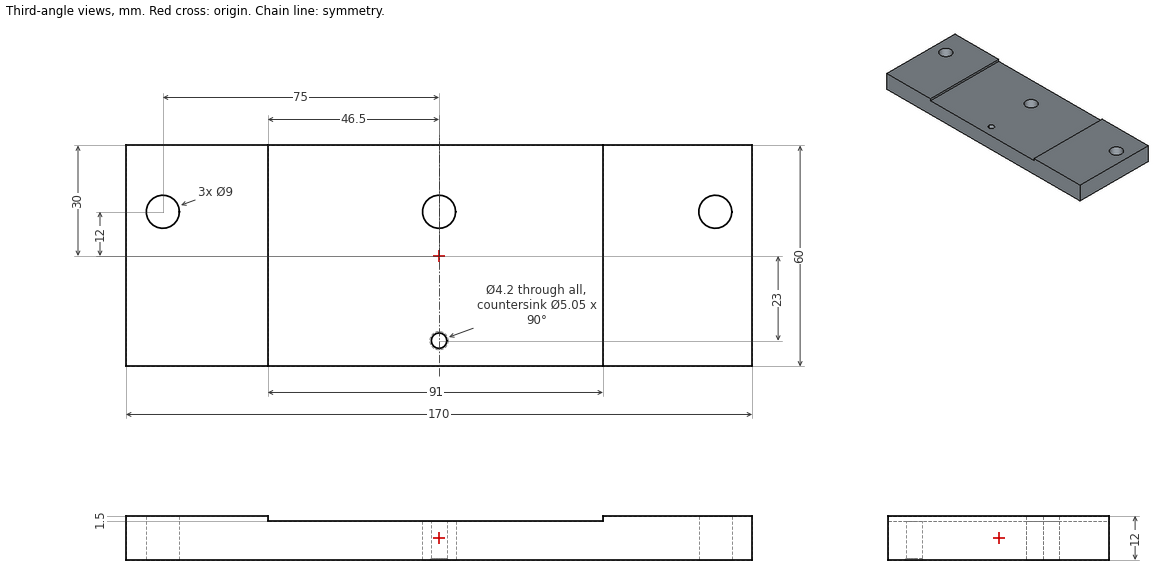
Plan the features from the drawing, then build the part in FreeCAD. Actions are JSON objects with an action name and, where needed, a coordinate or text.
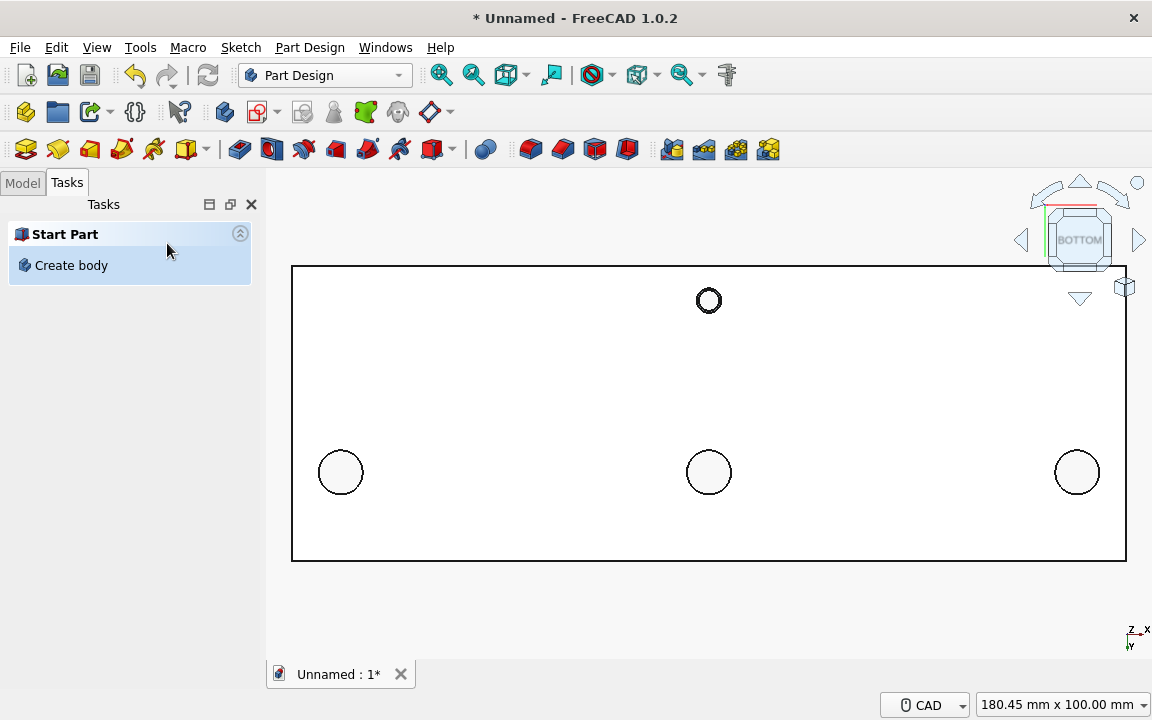
{"action": "key", "text": "0"}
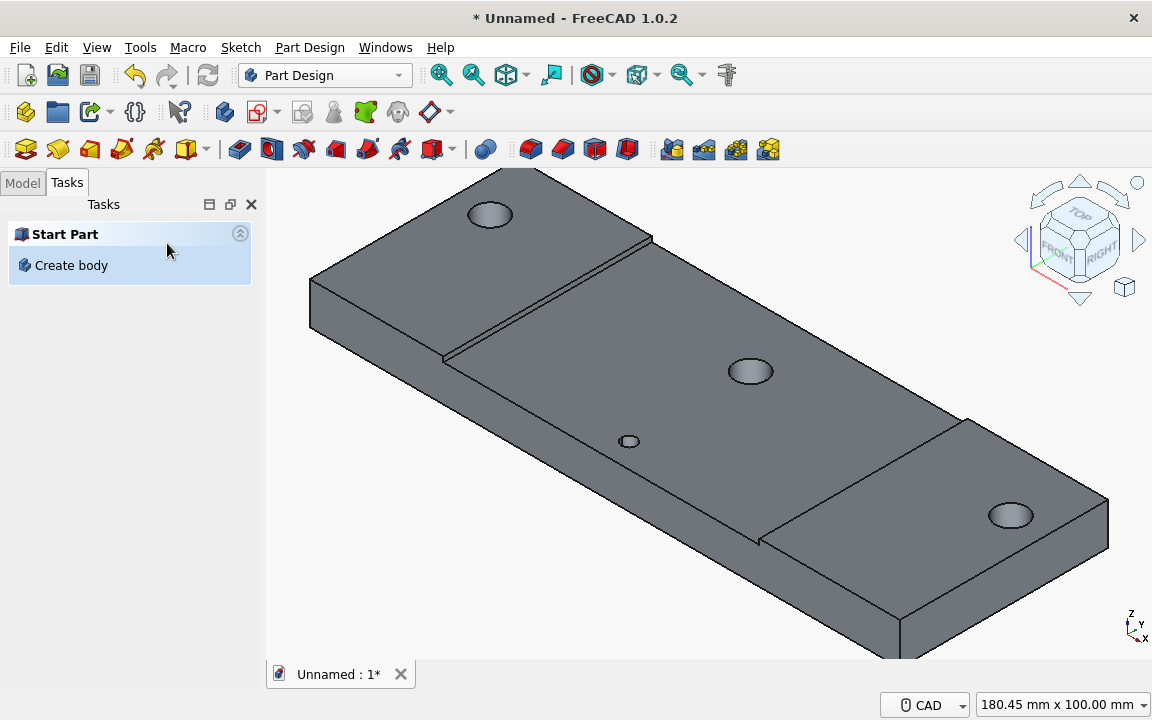
{"action": "key", "text": "v f"}